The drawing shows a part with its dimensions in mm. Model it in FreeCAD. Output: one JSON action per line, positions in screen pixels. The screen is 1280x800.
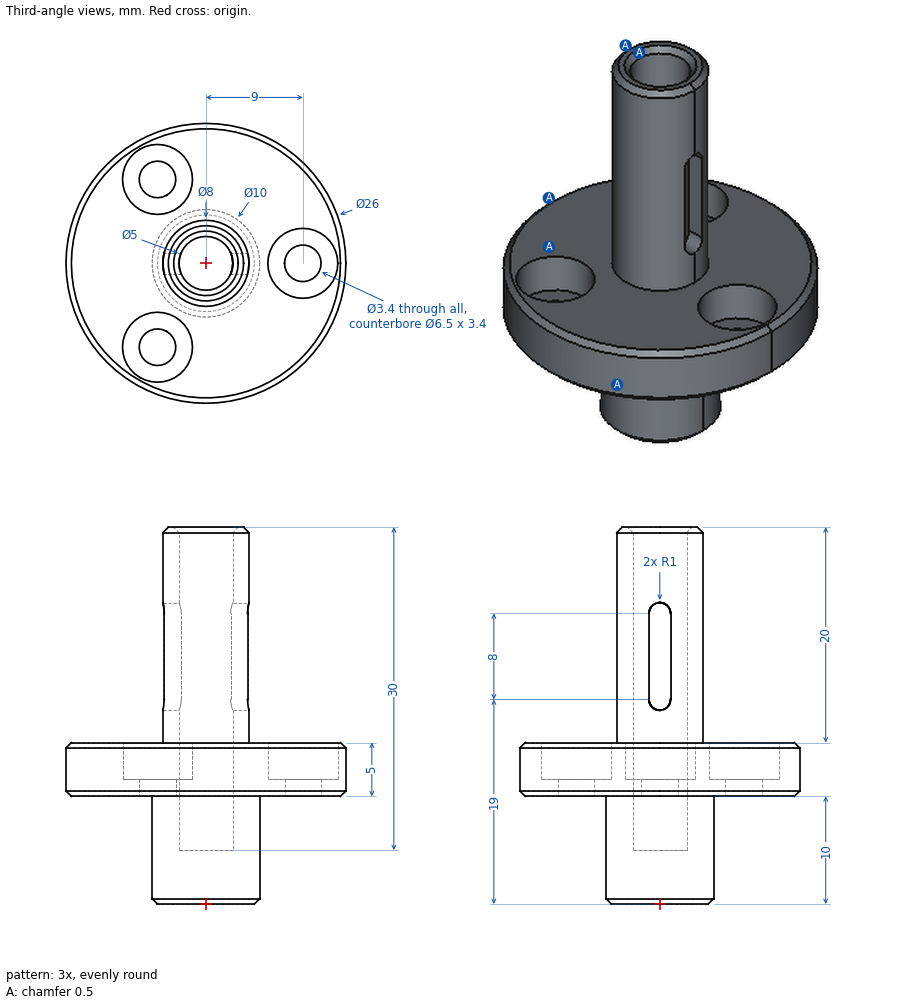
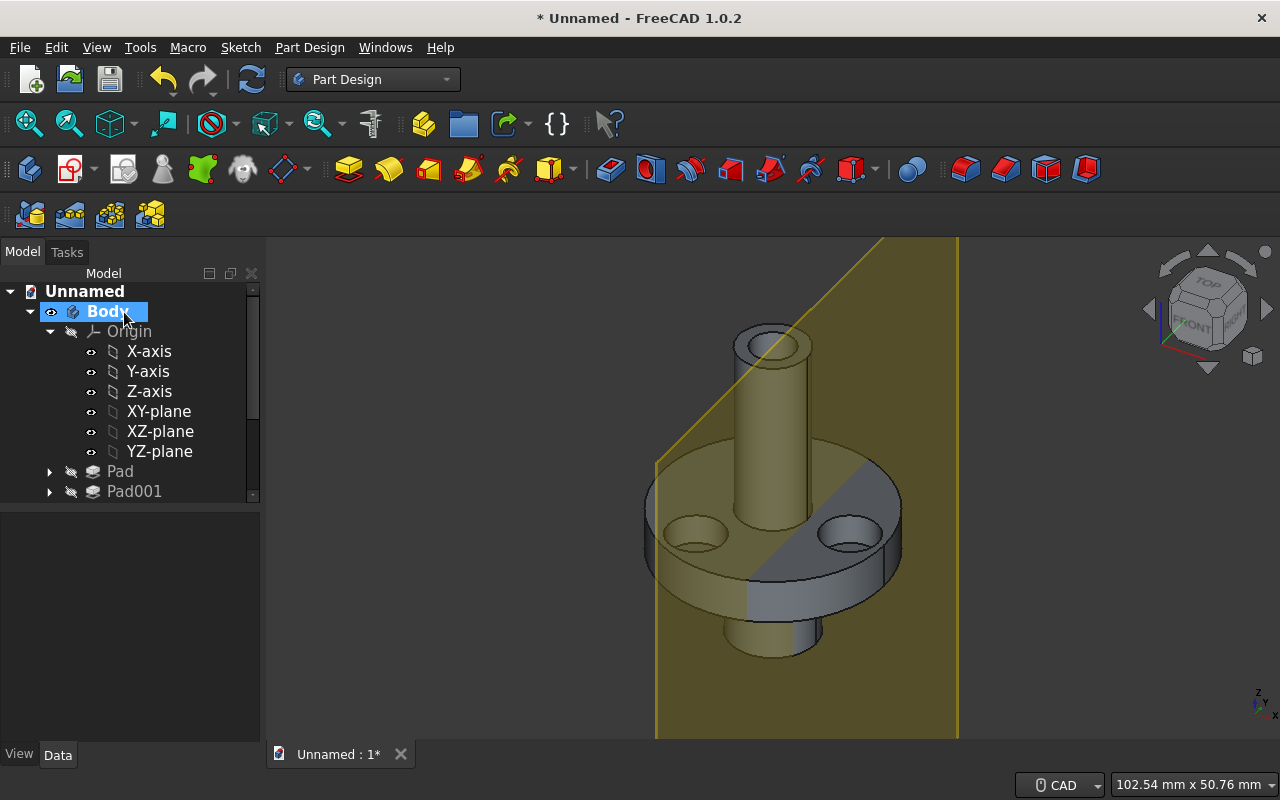
{"action": "scroll", "coordinate": [100, 387], "scroll_direction": "down", "scroll_amount": 3}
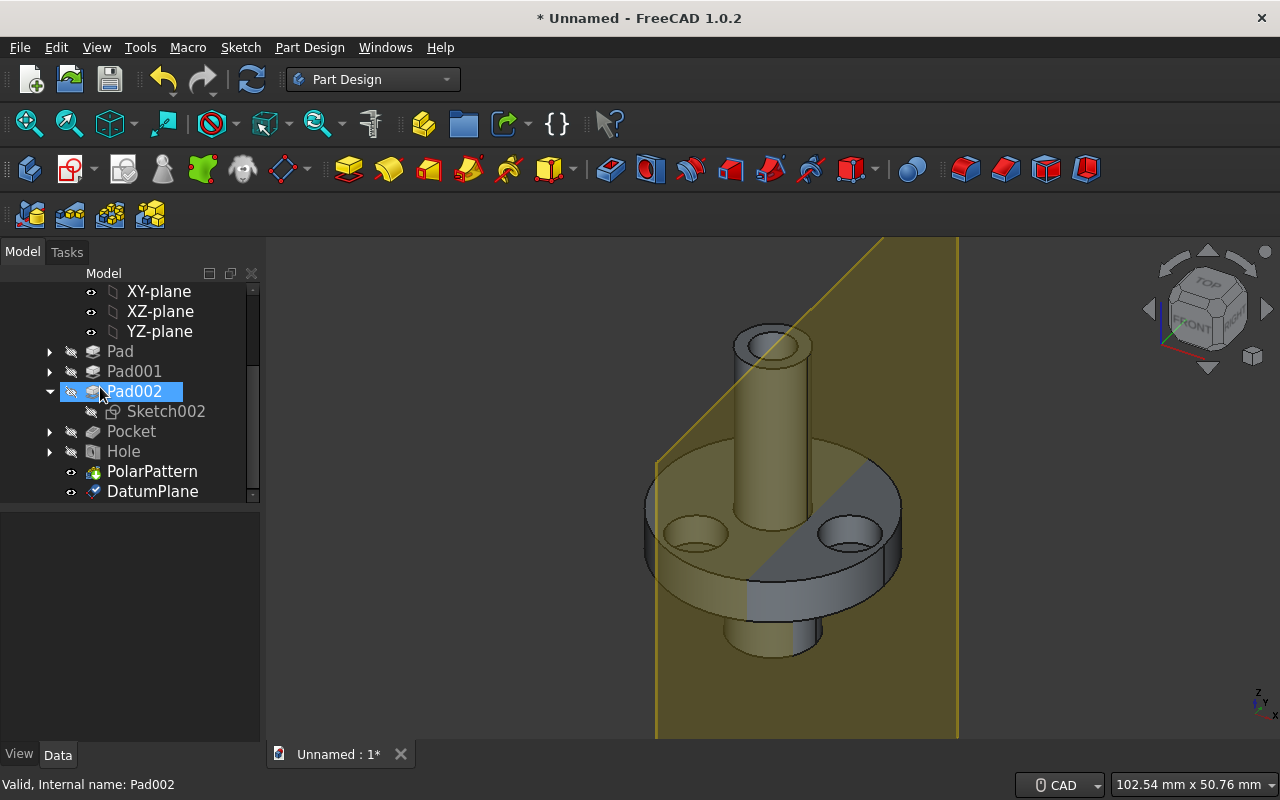
{"action": "left_click", "coordinate": [116, 492]}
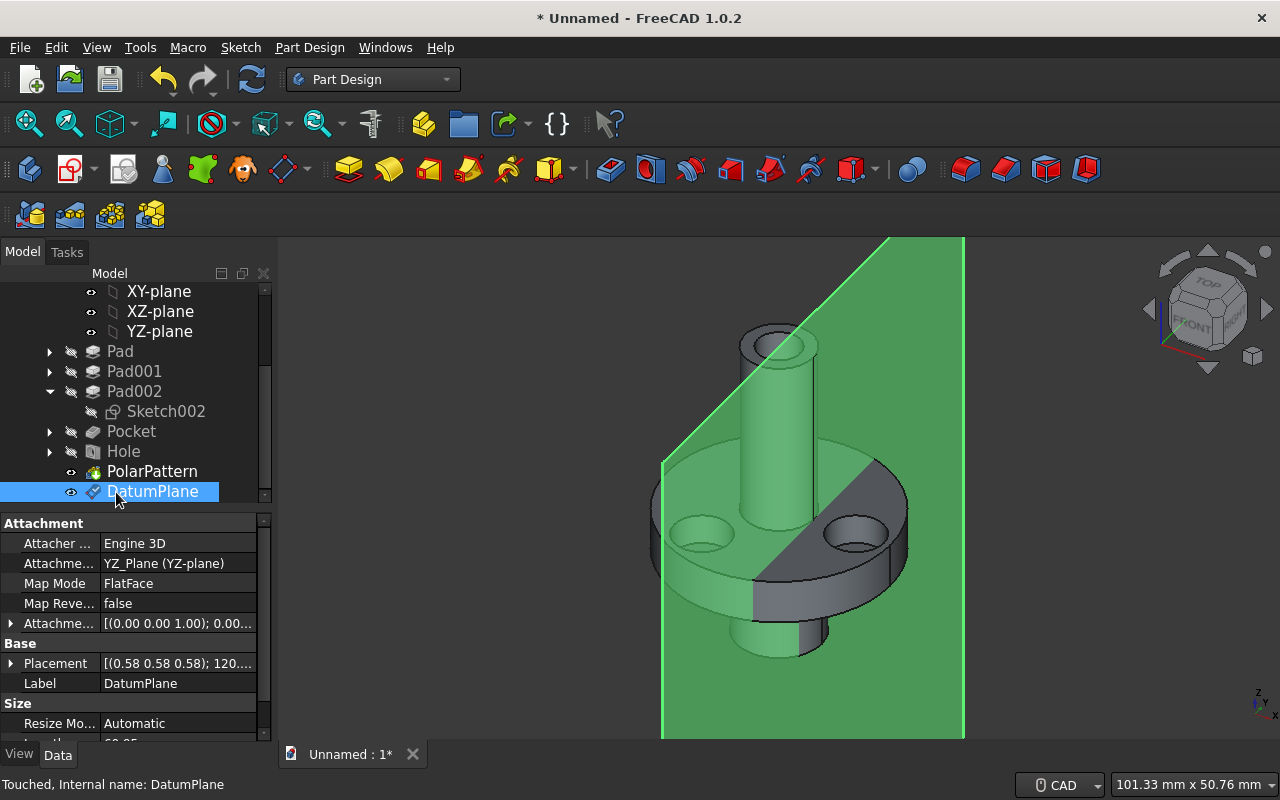
{"action": "left_click", "coordinate": [70, 170]}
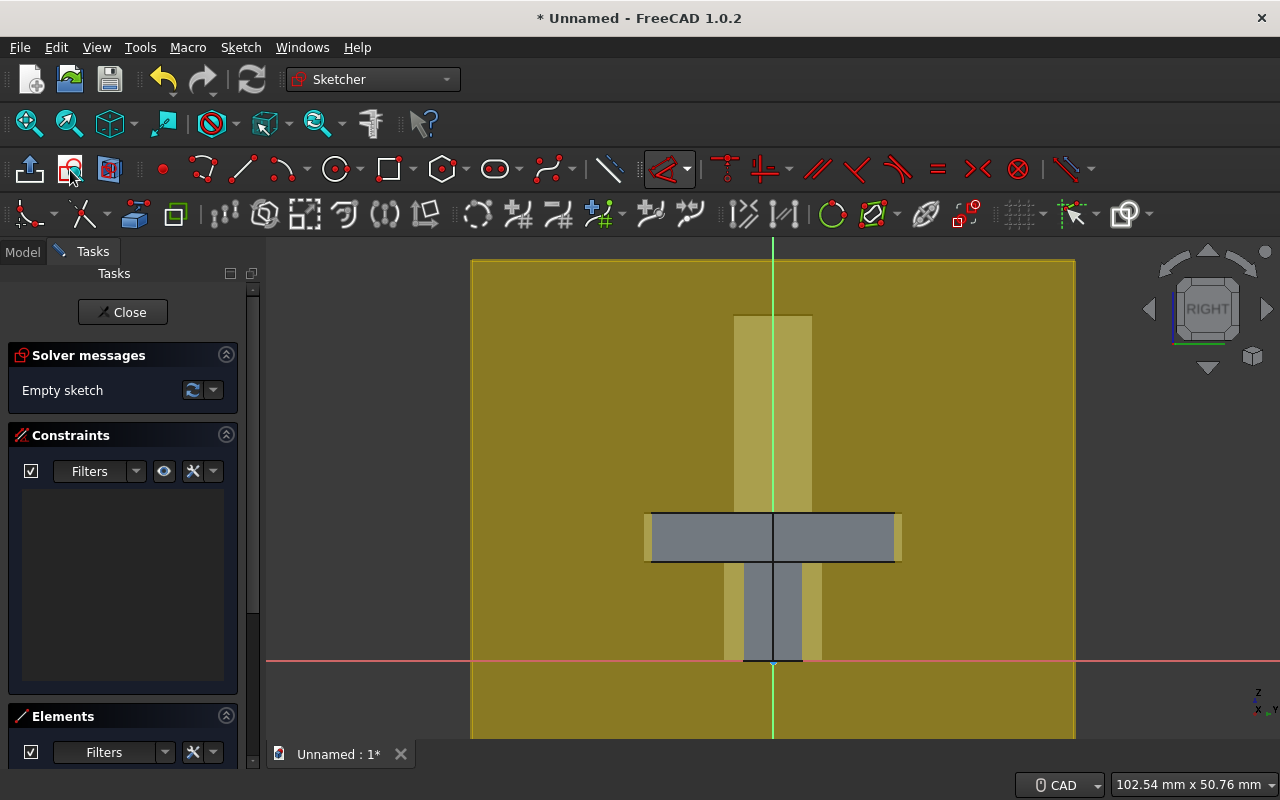
{"action": "left_click", "coordinate": [110, 170]}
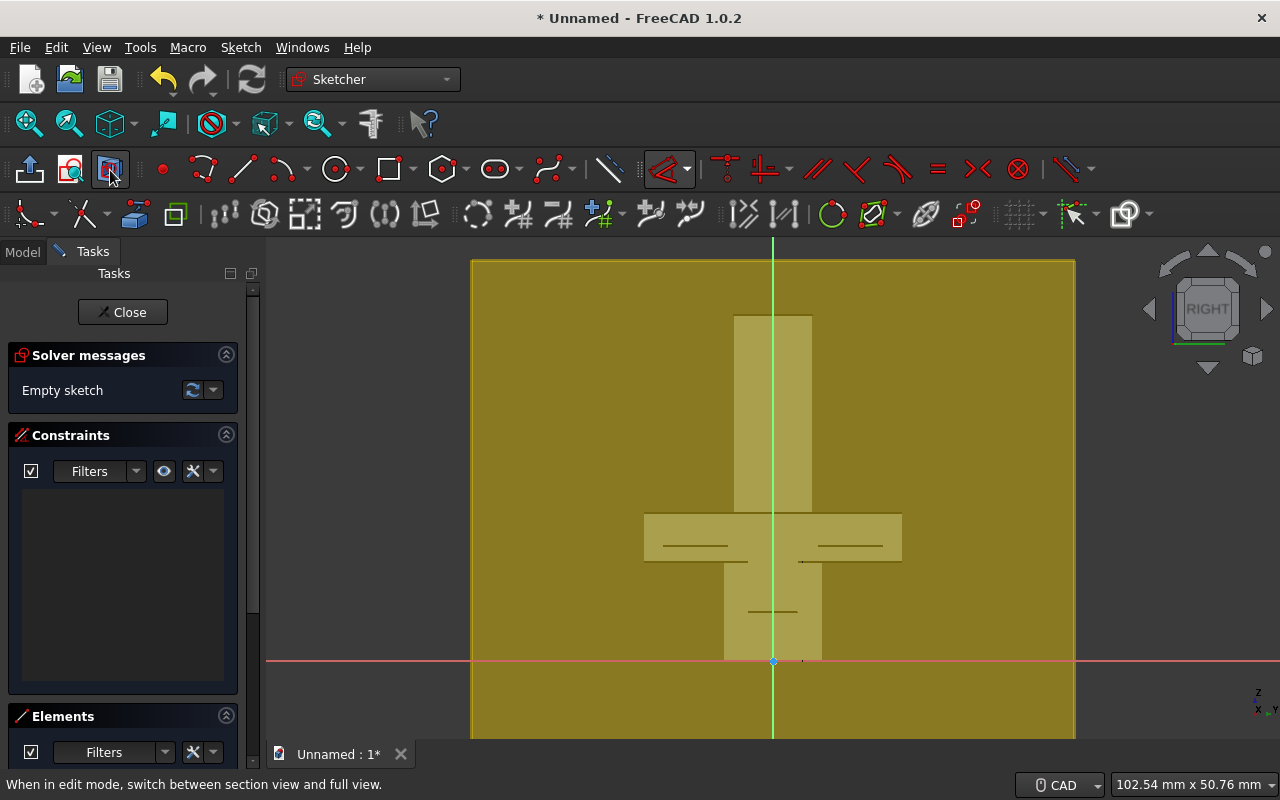
{"action": "scroll", "coordinate": [803, 410], "scroll_direction": "up", "scroll_amount": 6}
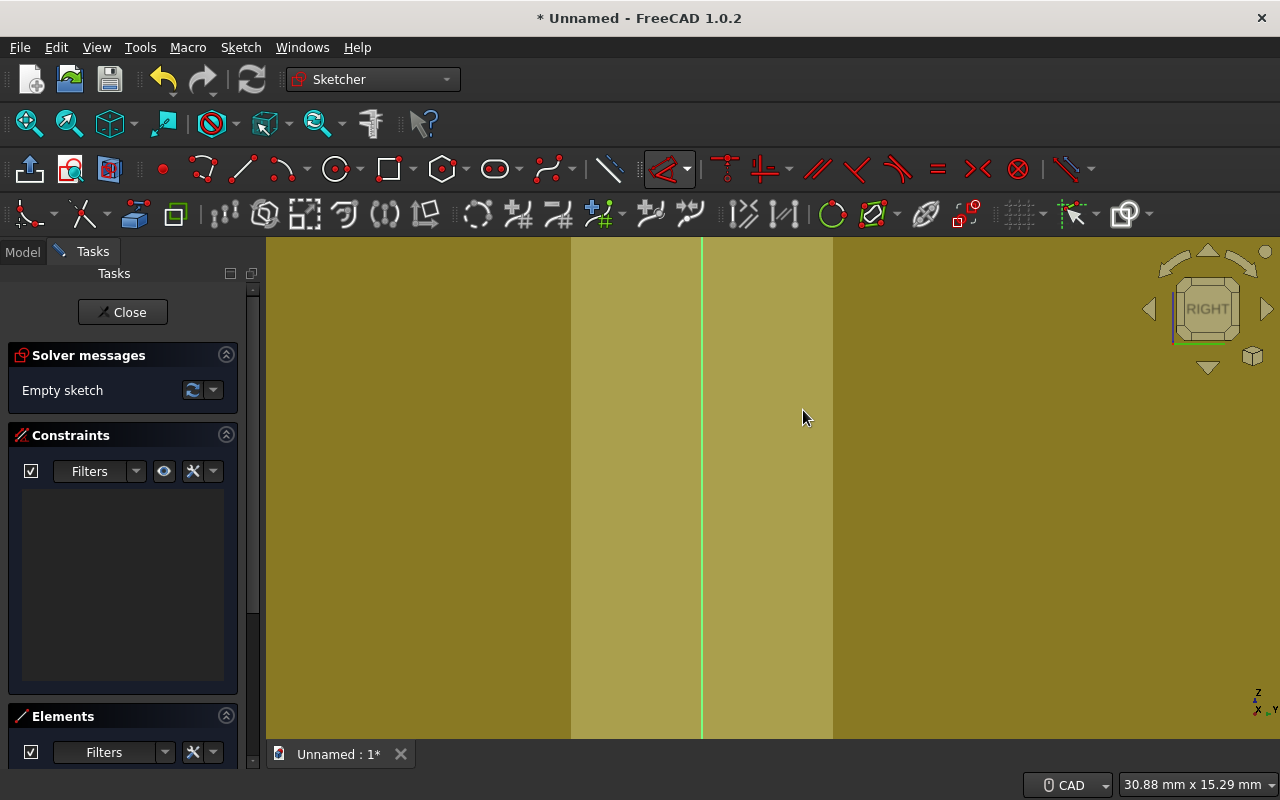
{"action": "left_click", "coordinate": [496, 170]}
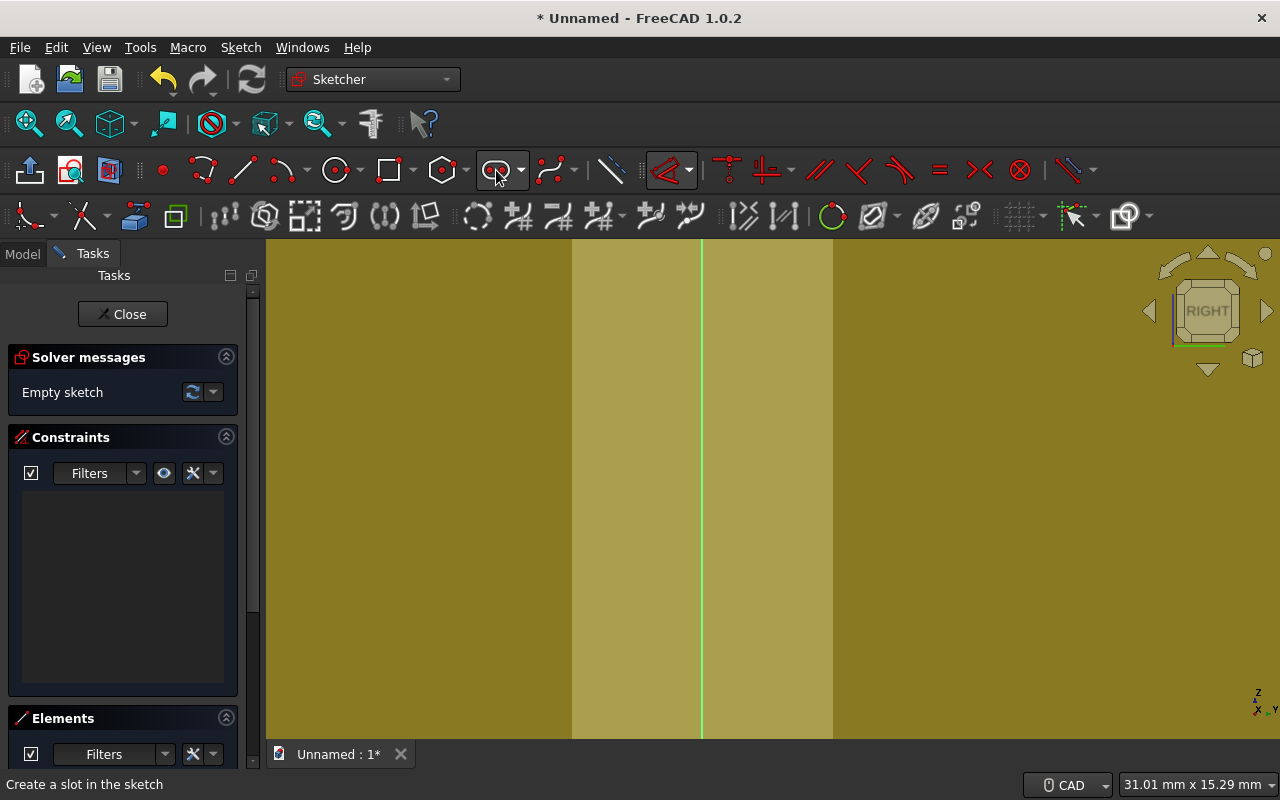
{"action": "left_click", "coordinate": [702, 619]}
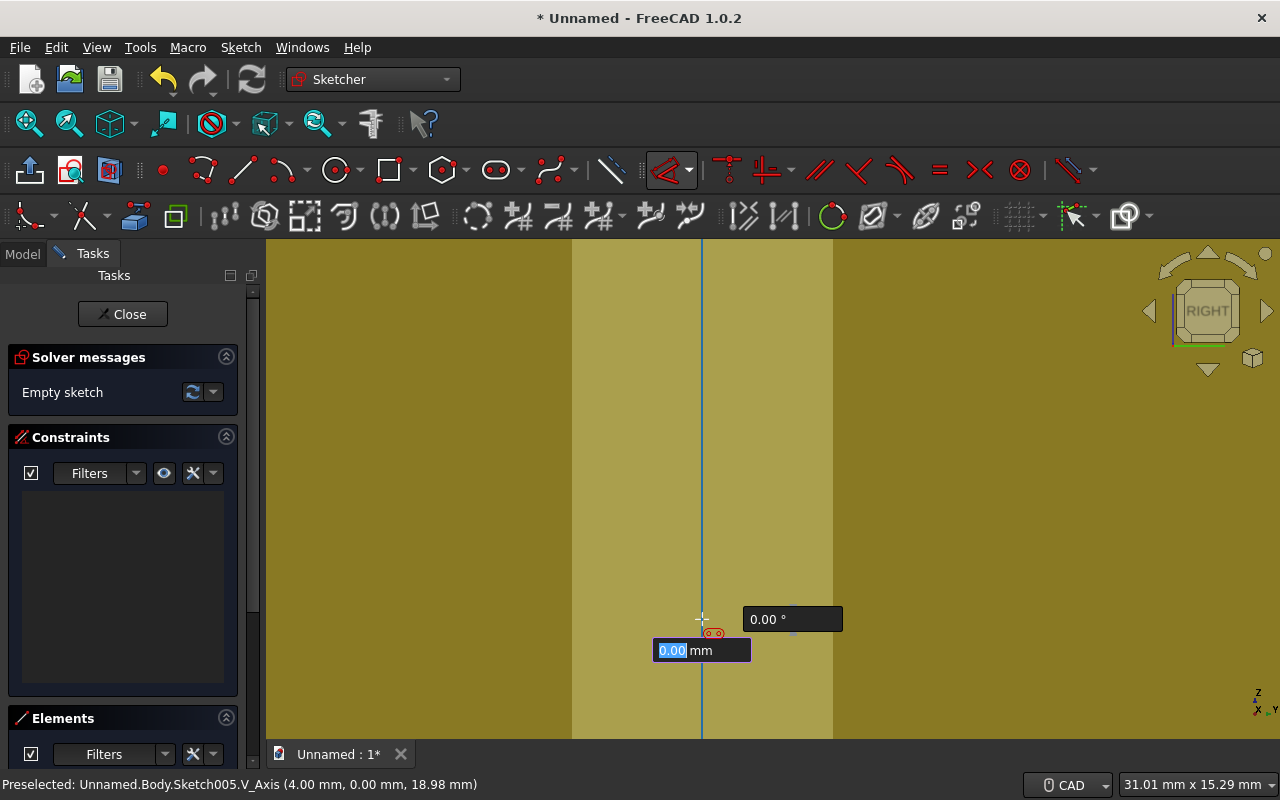
{"action": "left_click", "coordinate": [711, 358]}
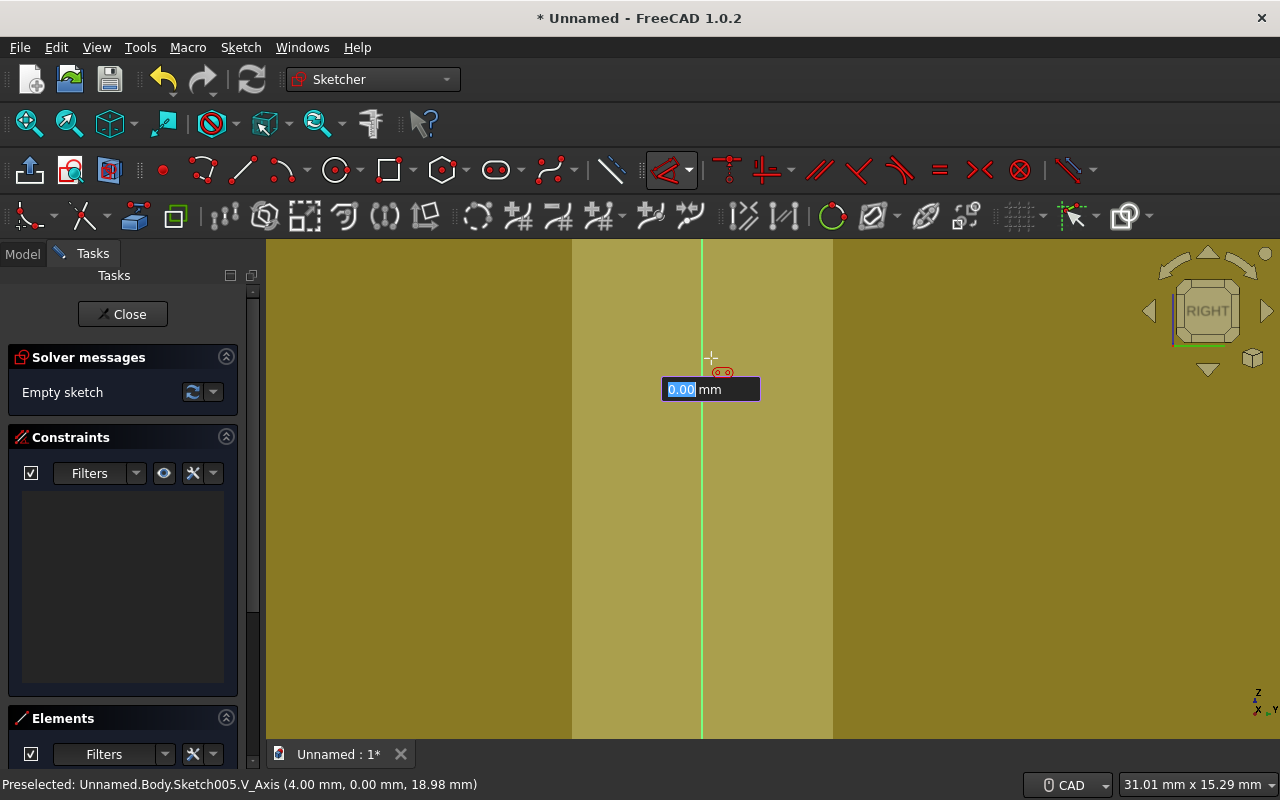
{"action": "left_click", "coordinate": [735, 489]}
{"action": "key", "text": "Escape"}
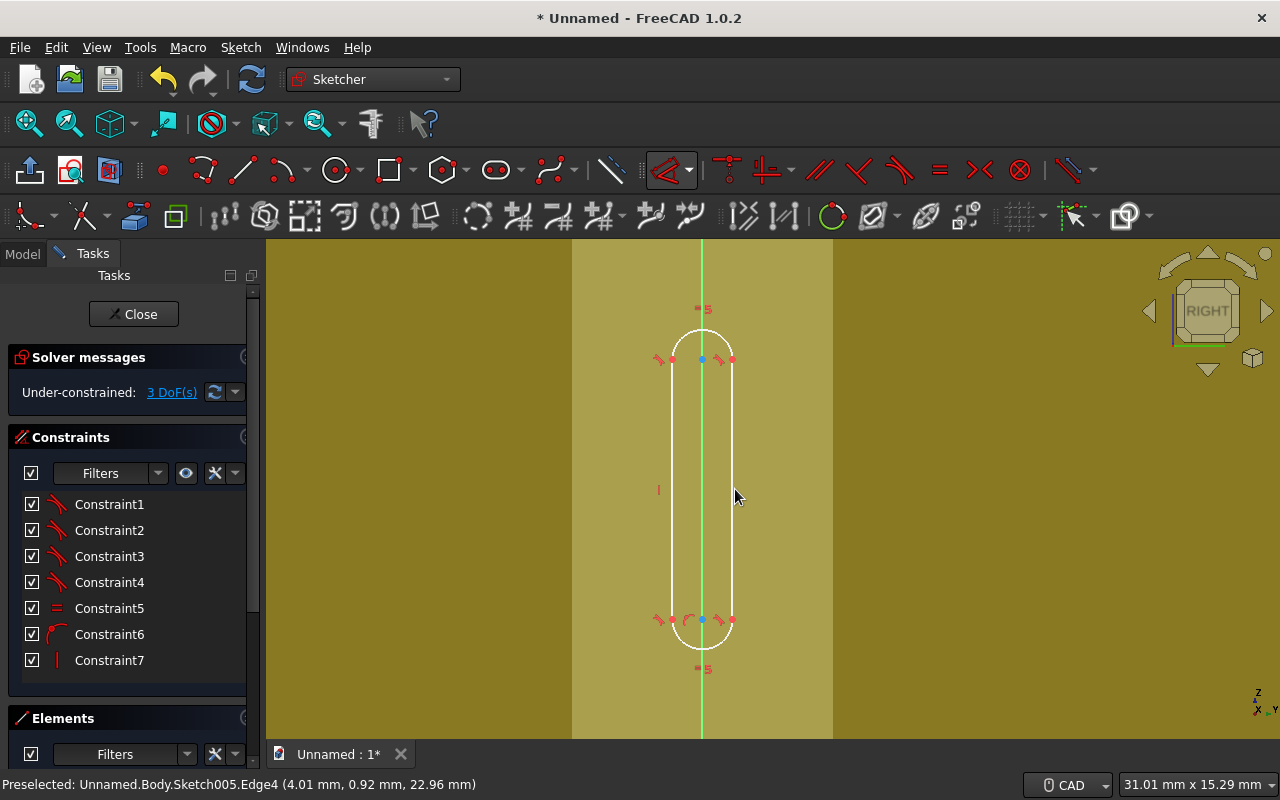
{"action": "left_click", "coordinate": [685, 644]}